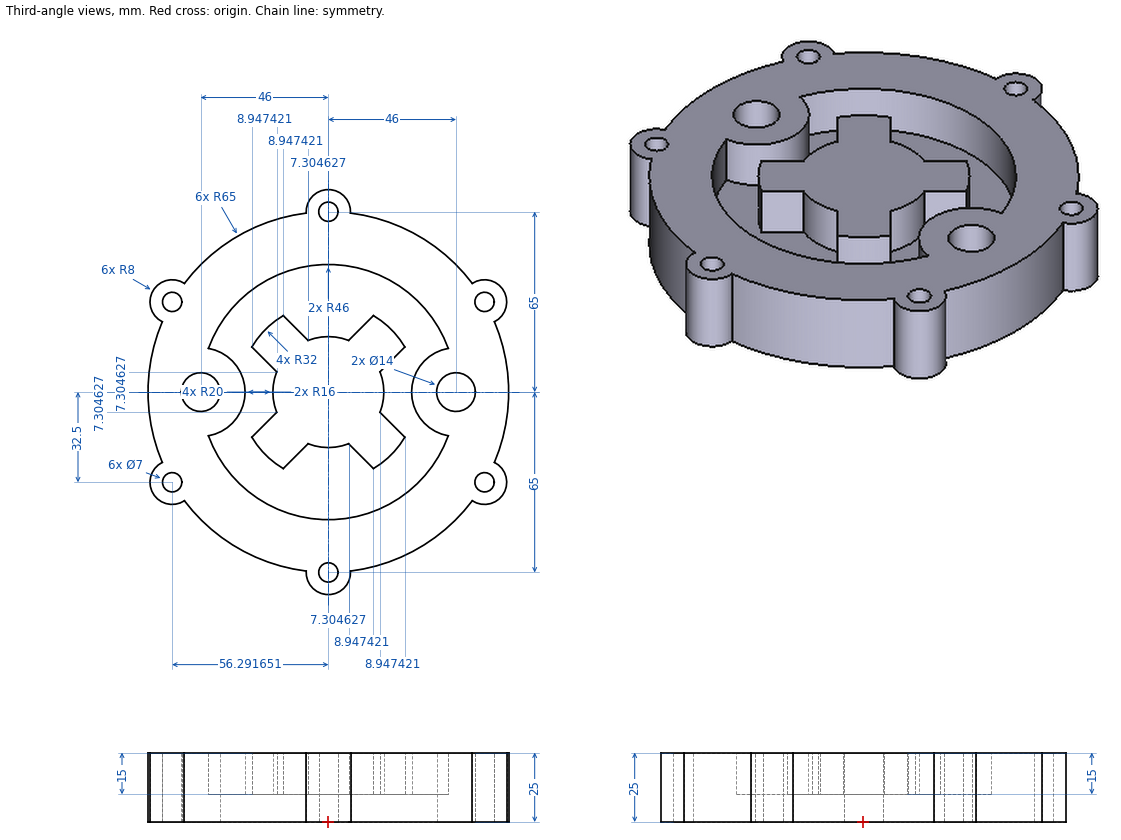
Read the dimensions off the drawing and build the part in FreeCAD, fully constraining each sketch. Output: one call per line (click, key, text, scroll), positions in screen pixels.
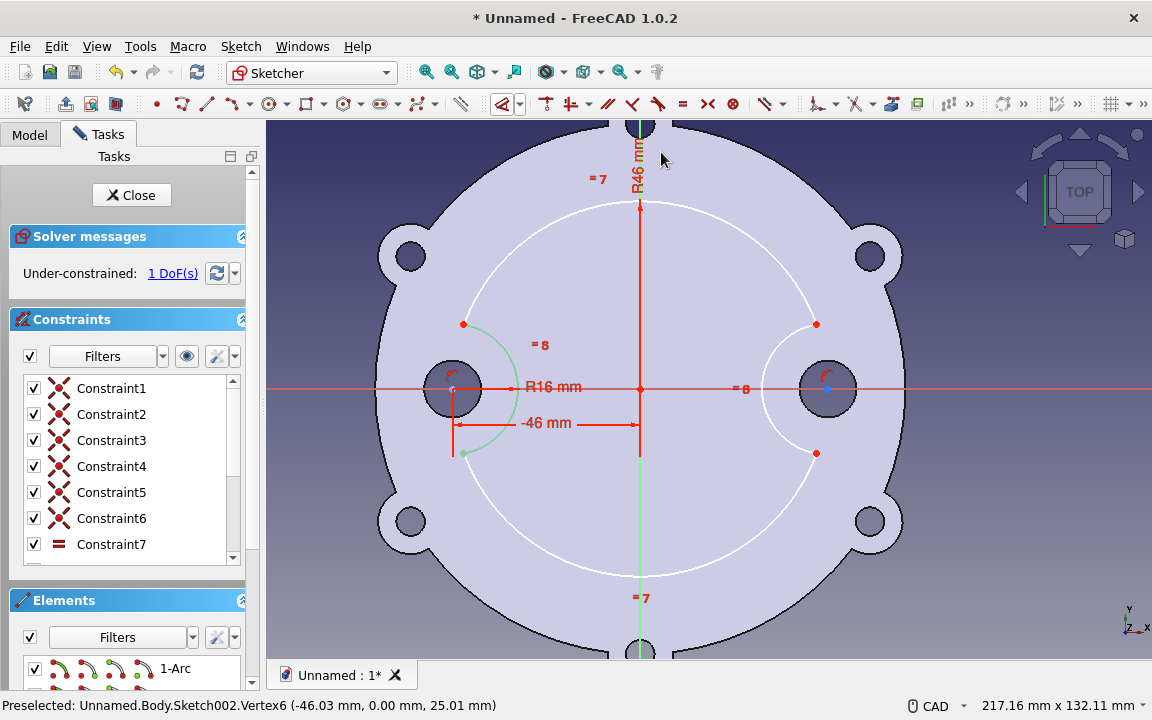
click(827, 389)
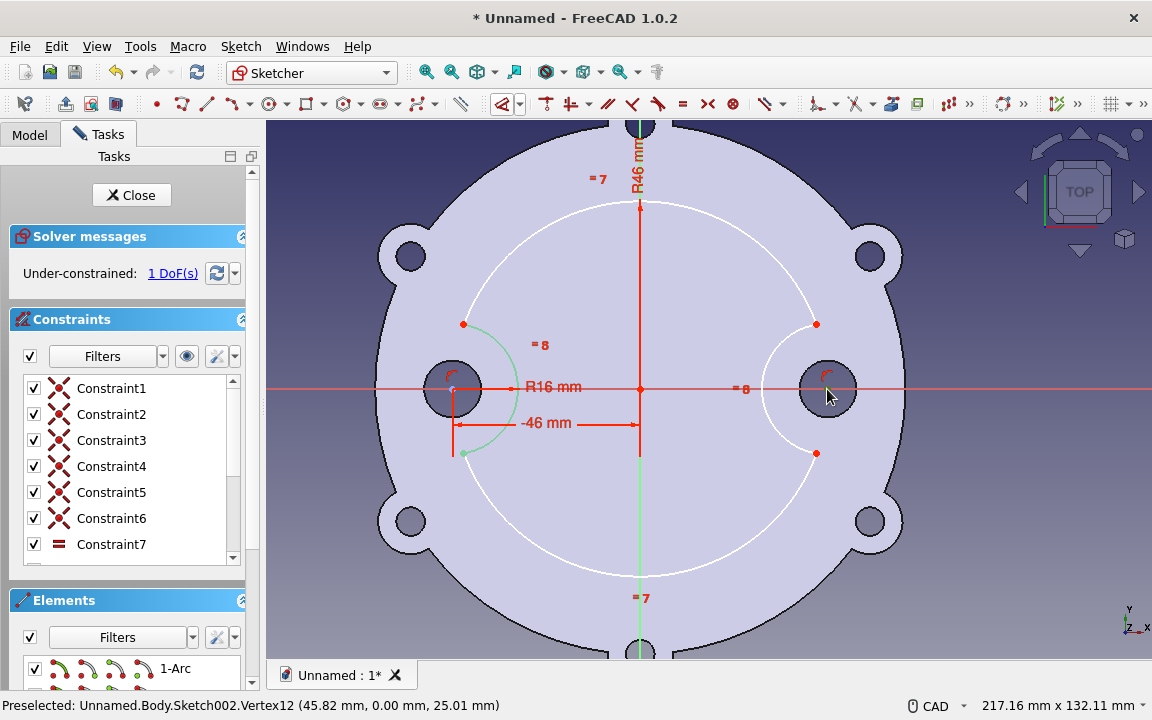
key(l)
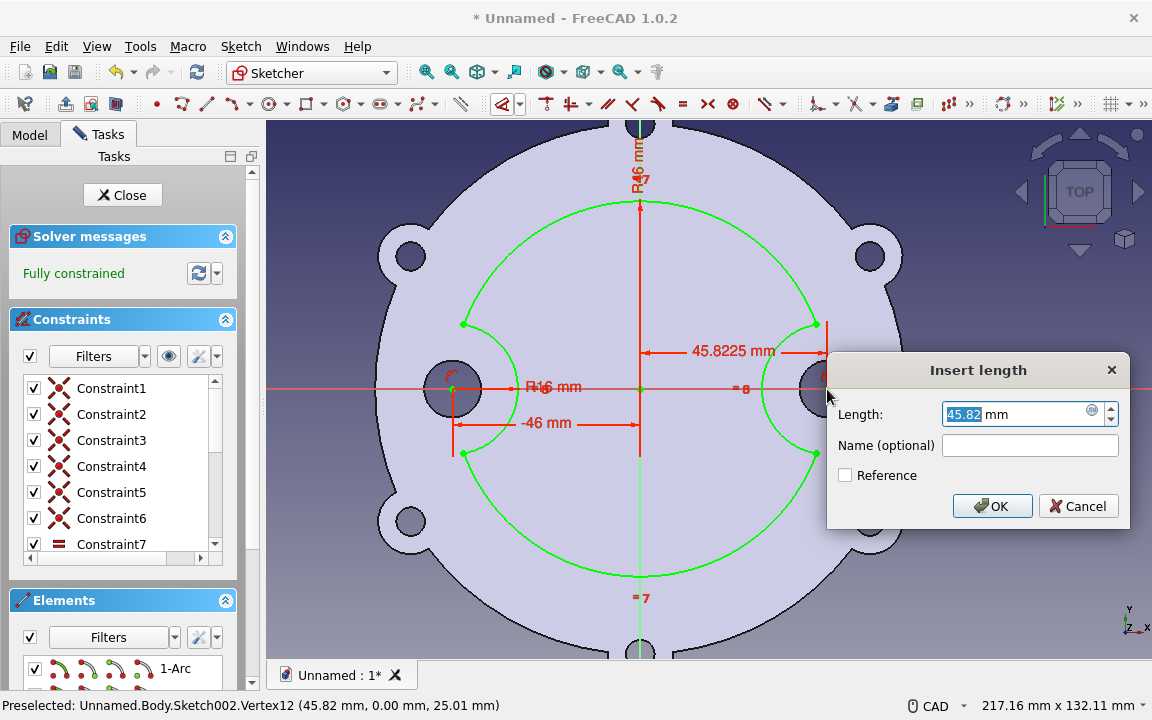
text(46)
key(Return)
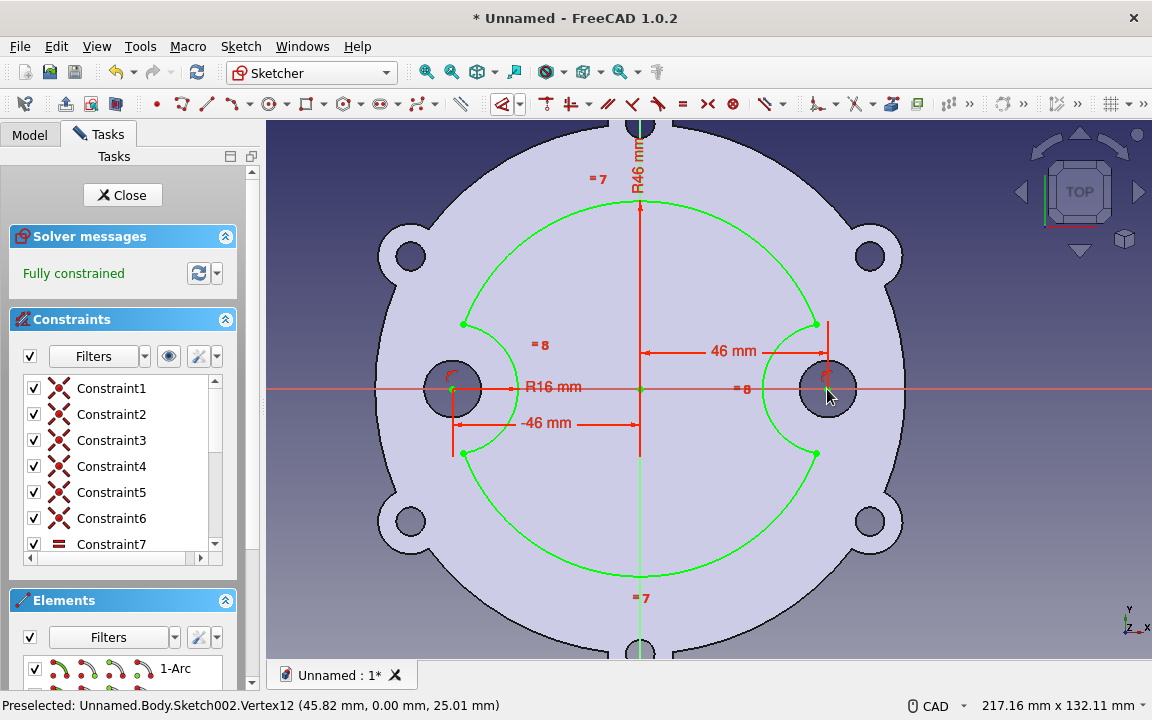
click(123, 195)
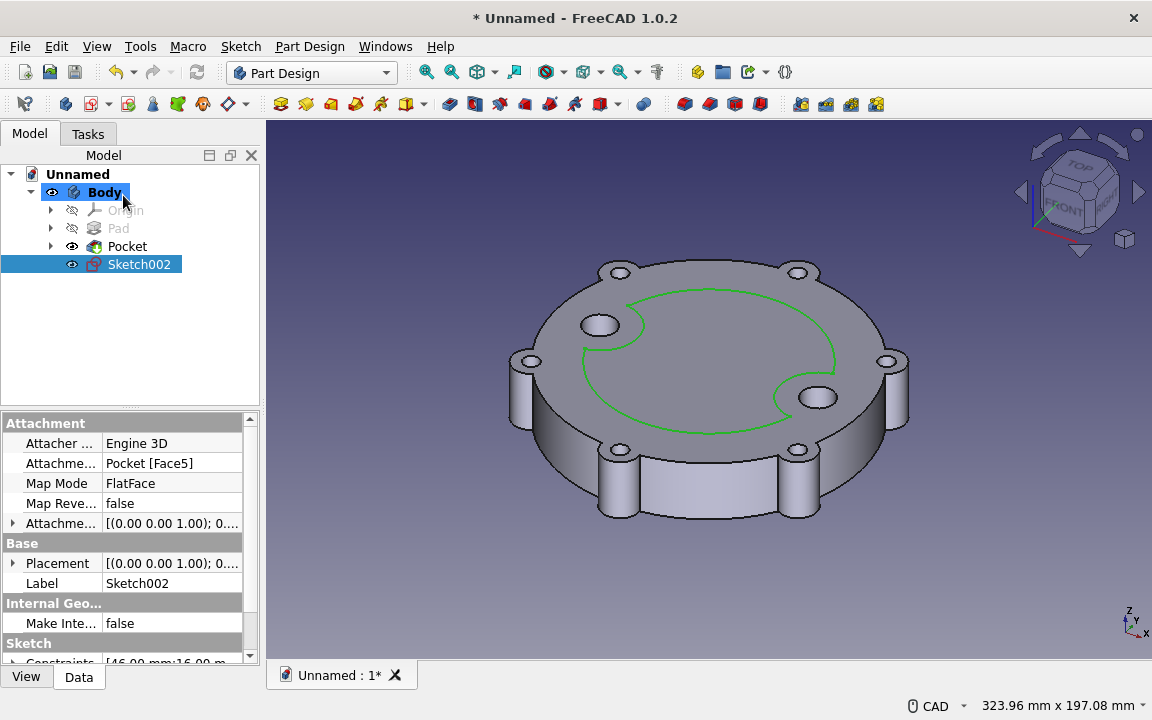
click(450, 104)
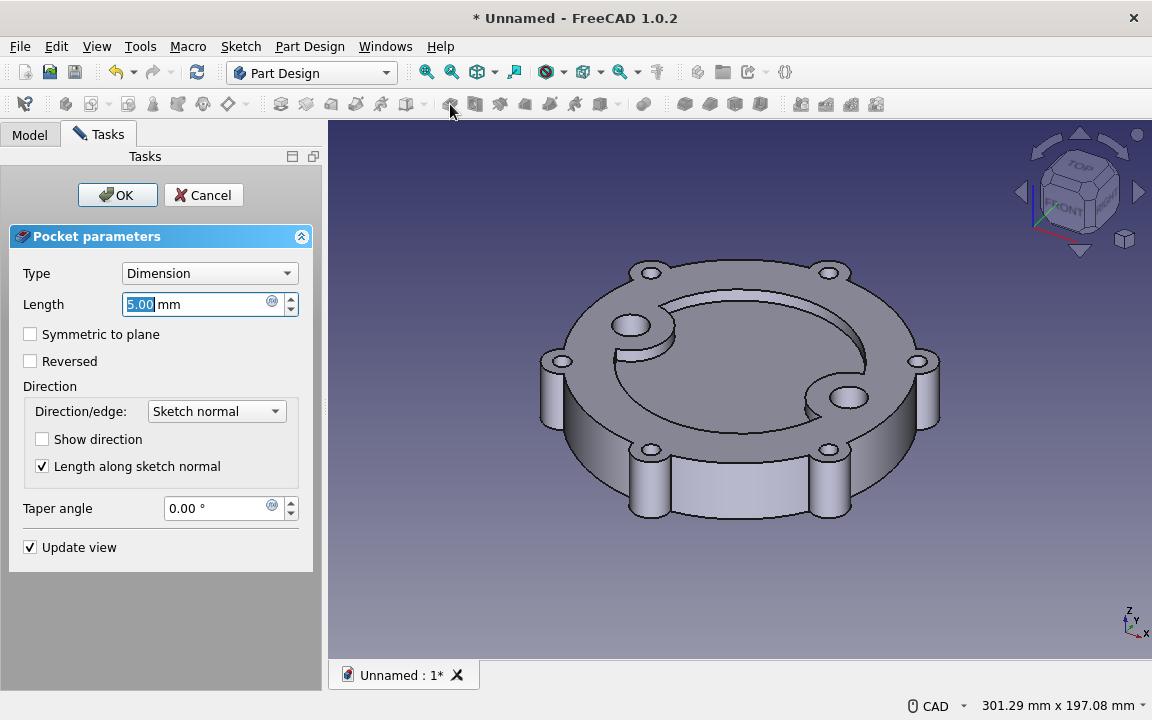
text(15)
key(Tab)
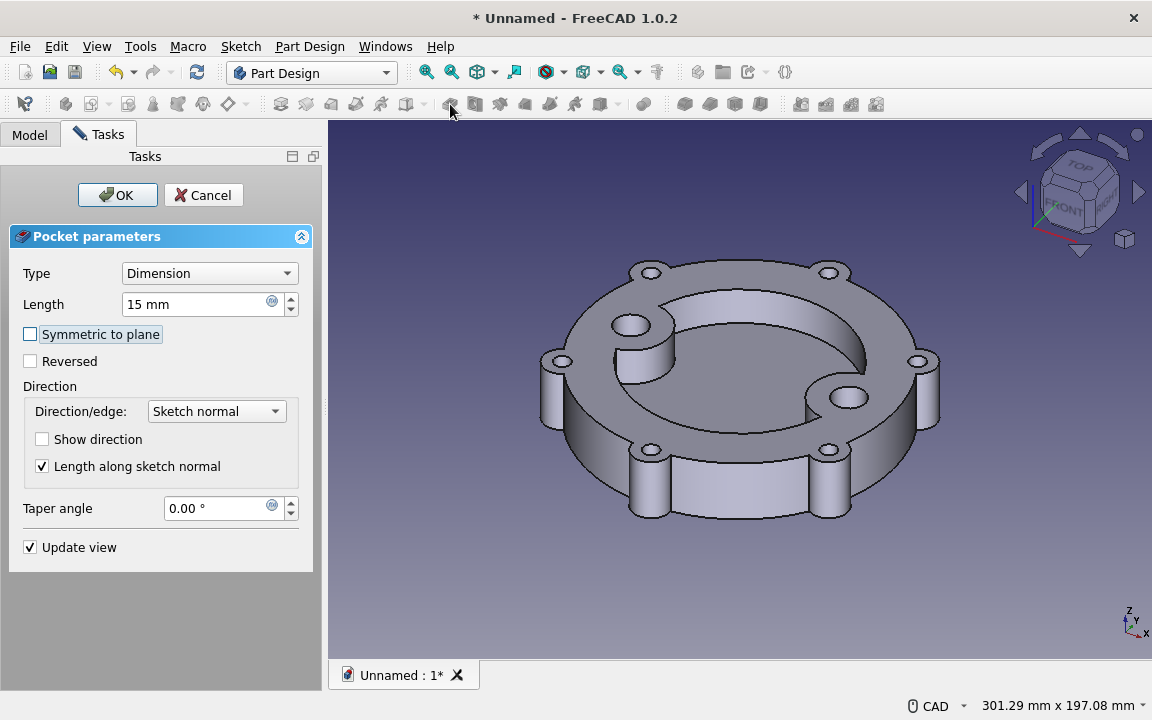
click(118, 195)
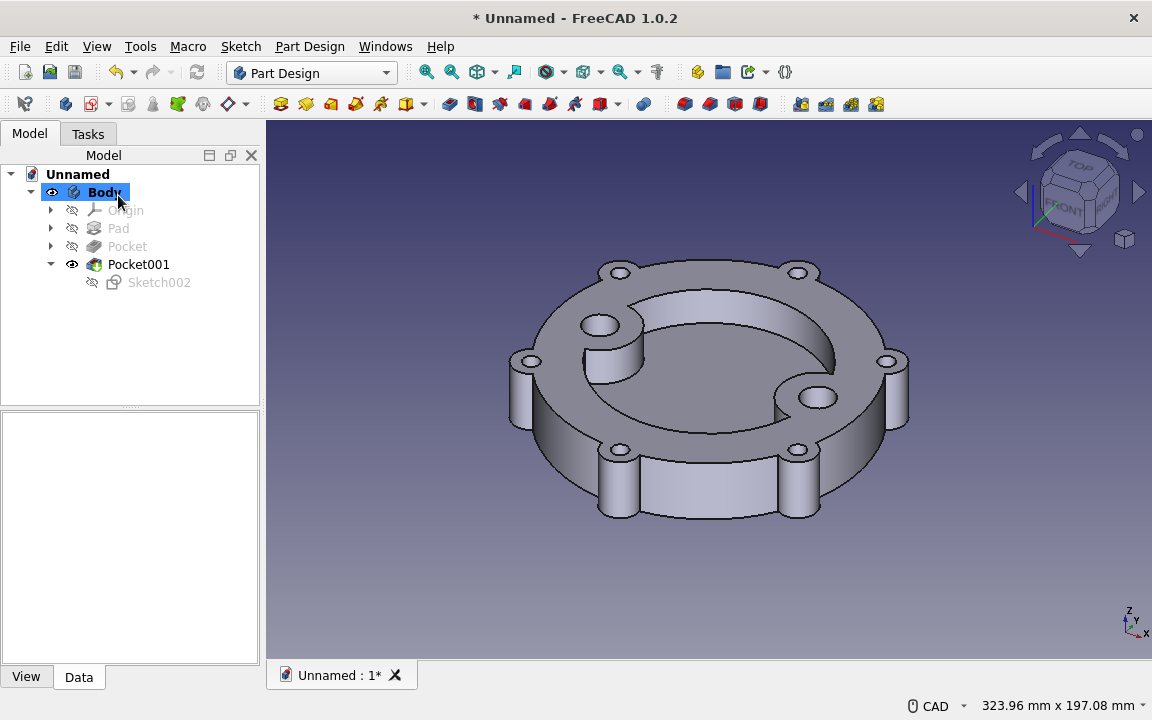
click(691, 412)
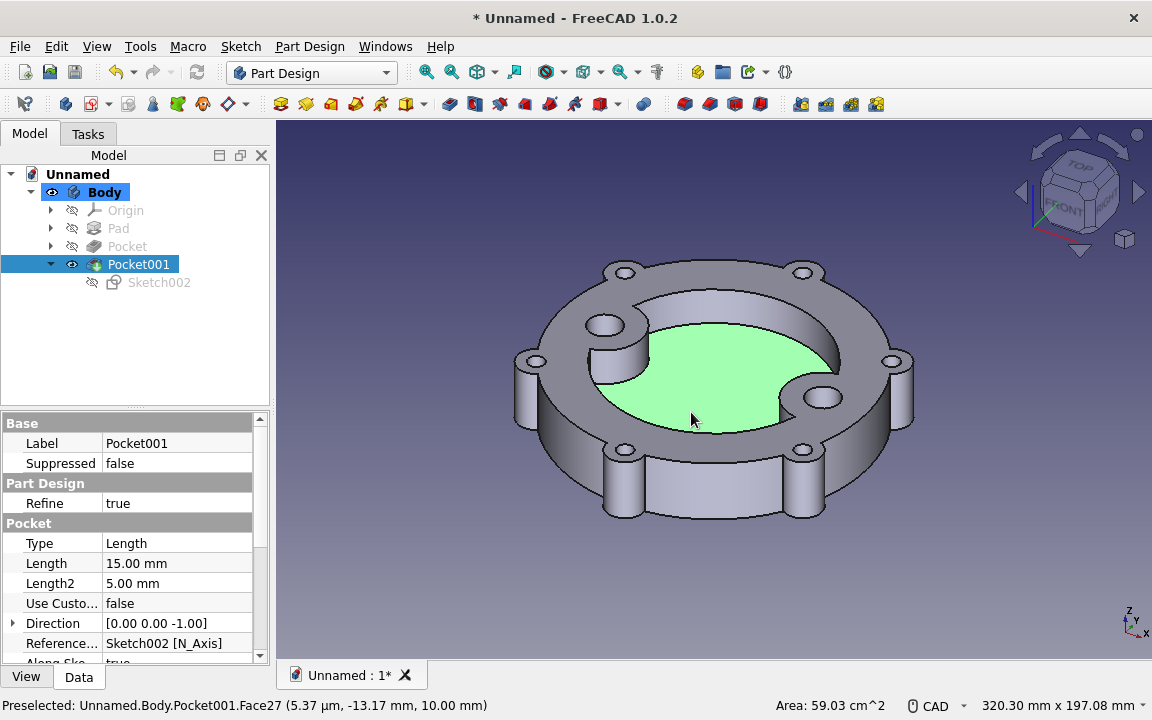
click(90, 104)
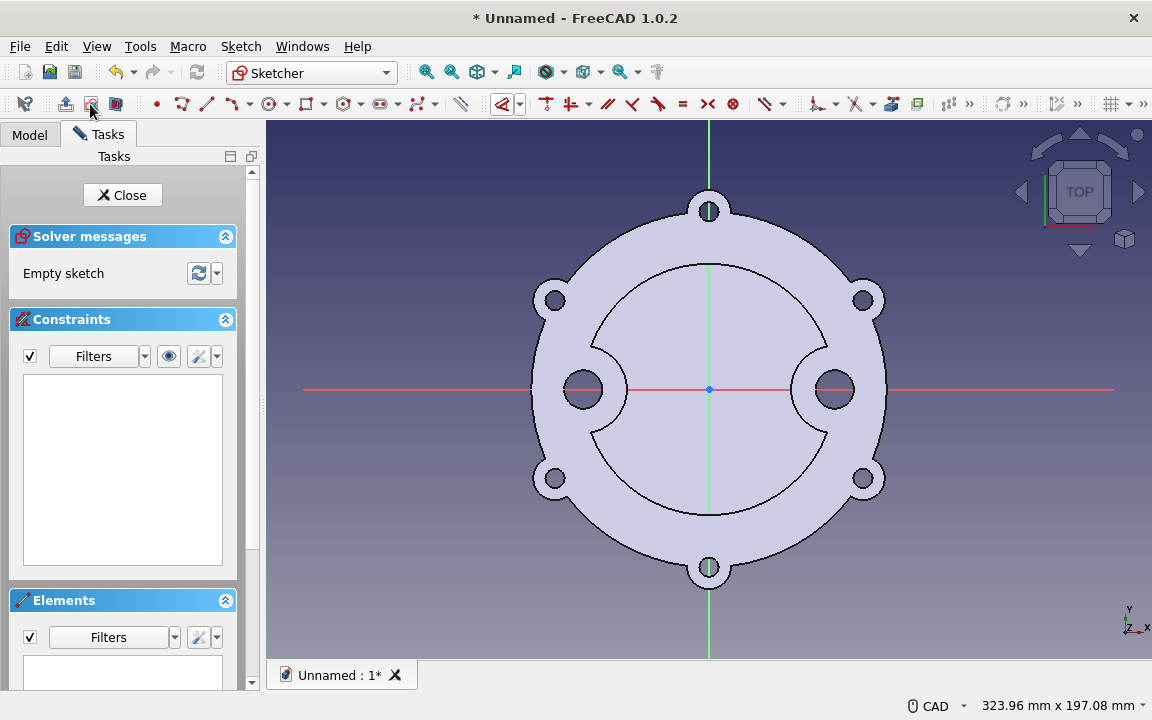
click(116, 104)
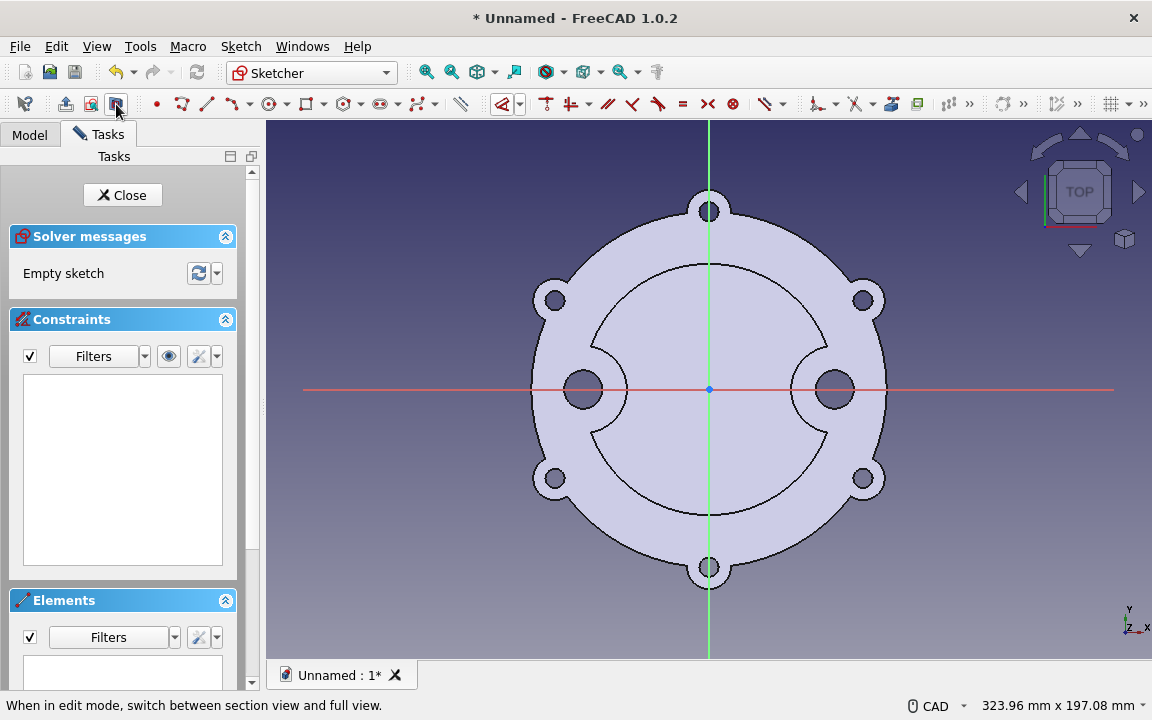
scroll(765, 390, up, 4)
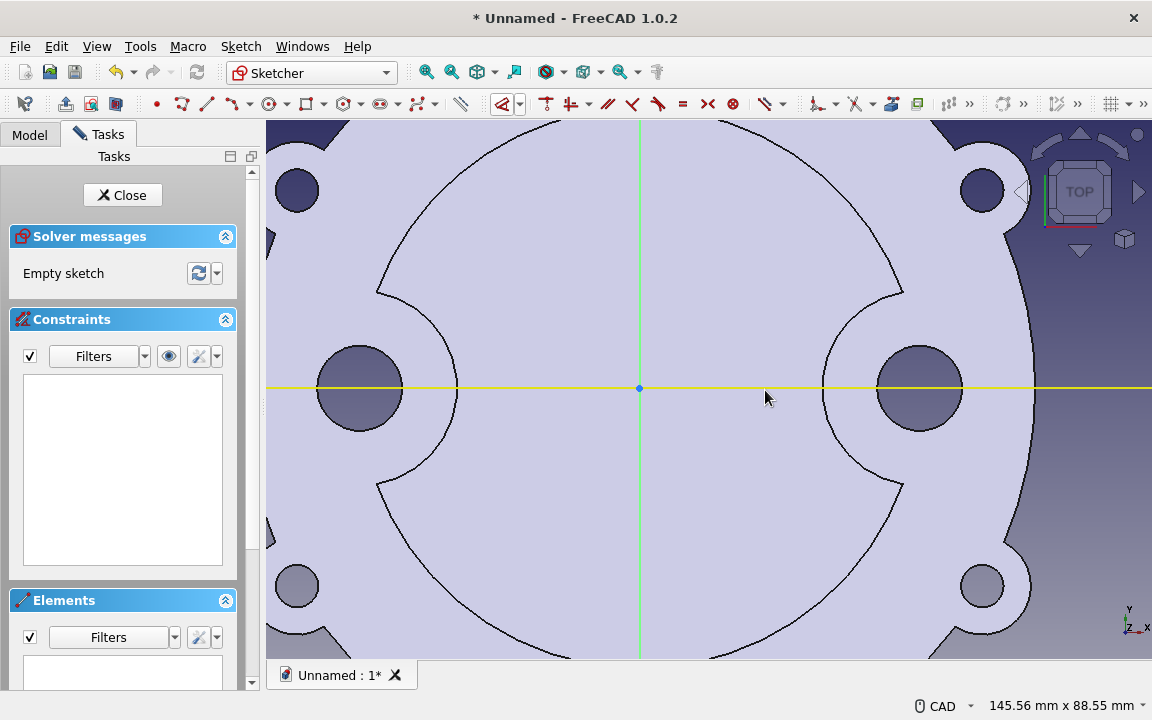
click(207, 104)